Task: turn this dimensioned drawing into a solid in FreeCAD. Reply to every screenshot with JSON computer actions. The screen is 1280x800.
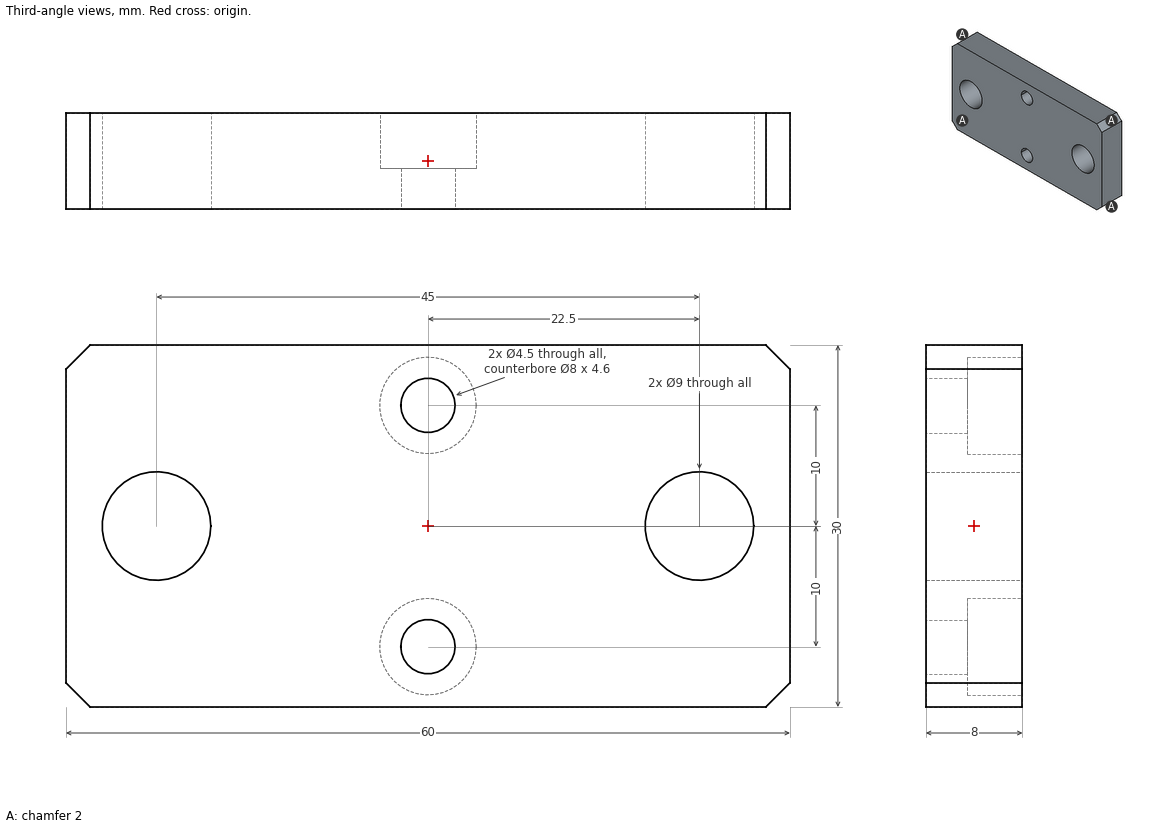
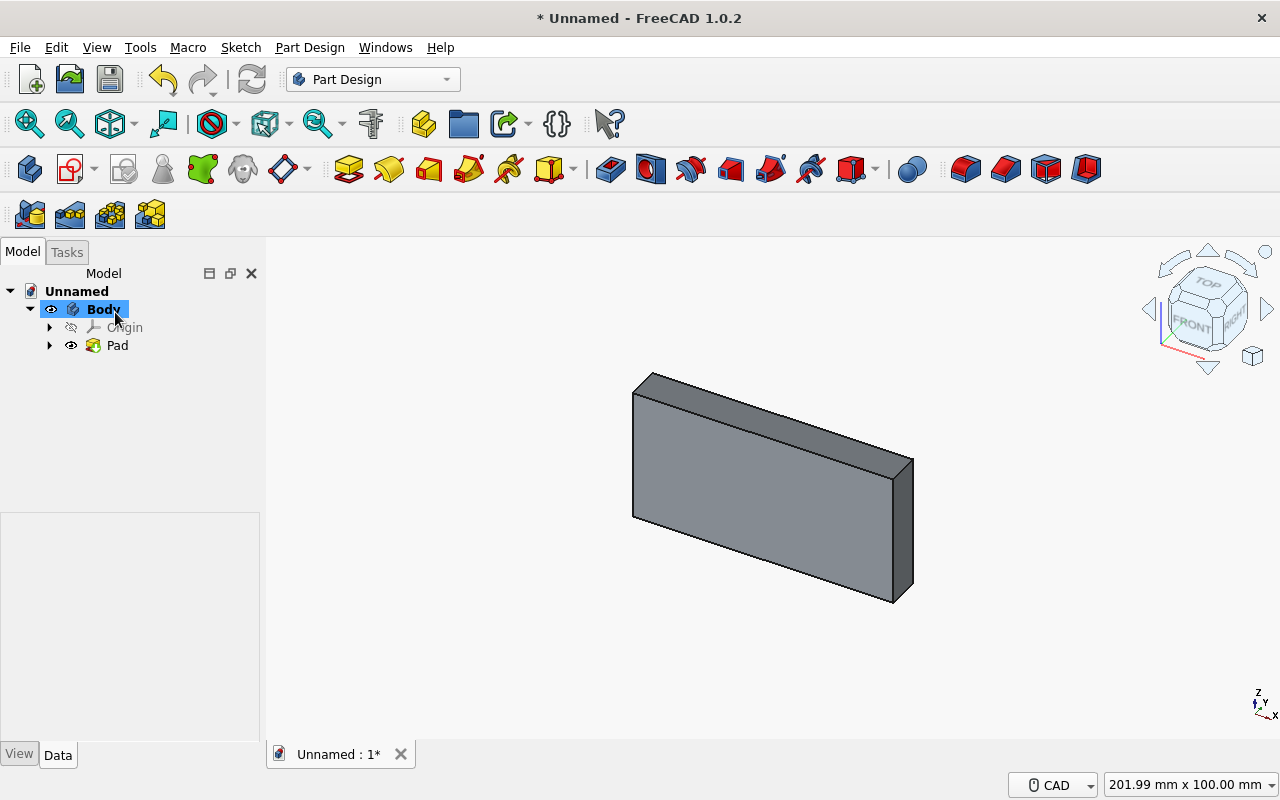
{"action": "left_click", "coordinate": [903, 469]}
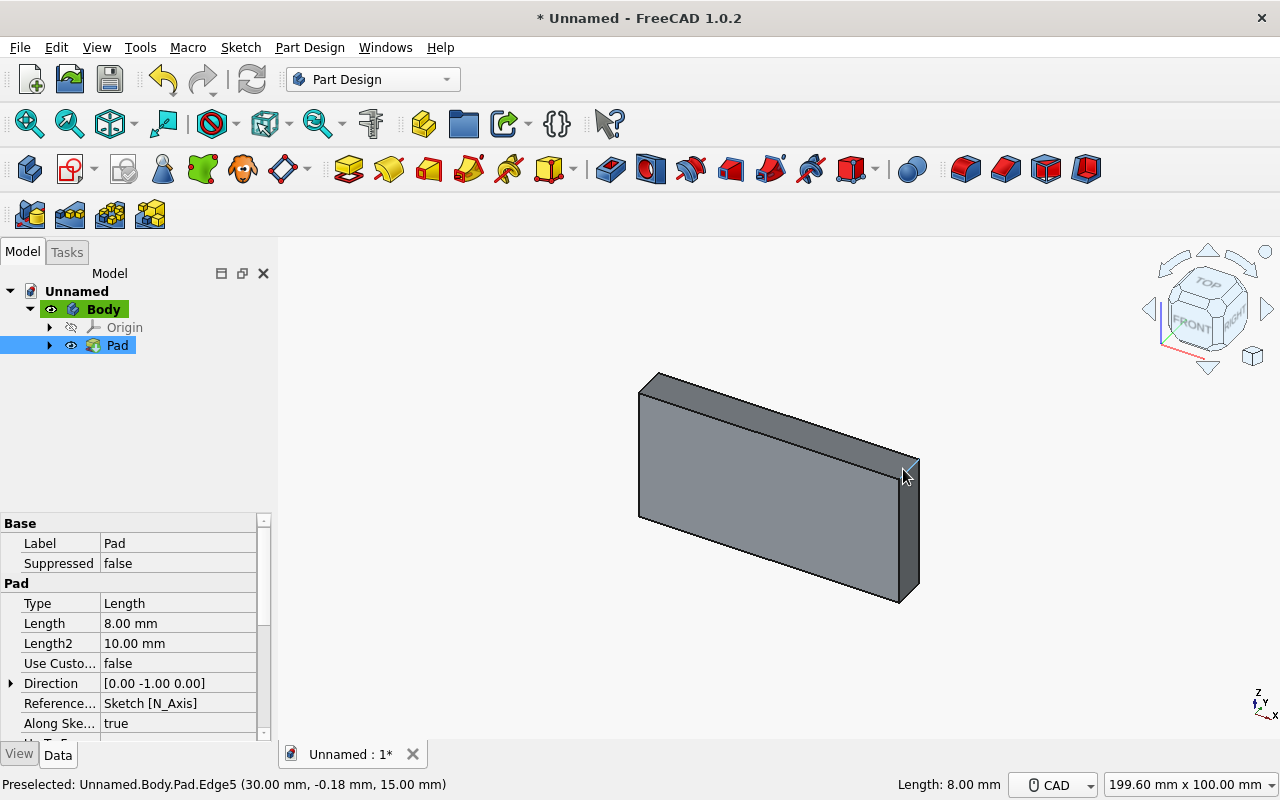
{"action": "key", "text": "0"}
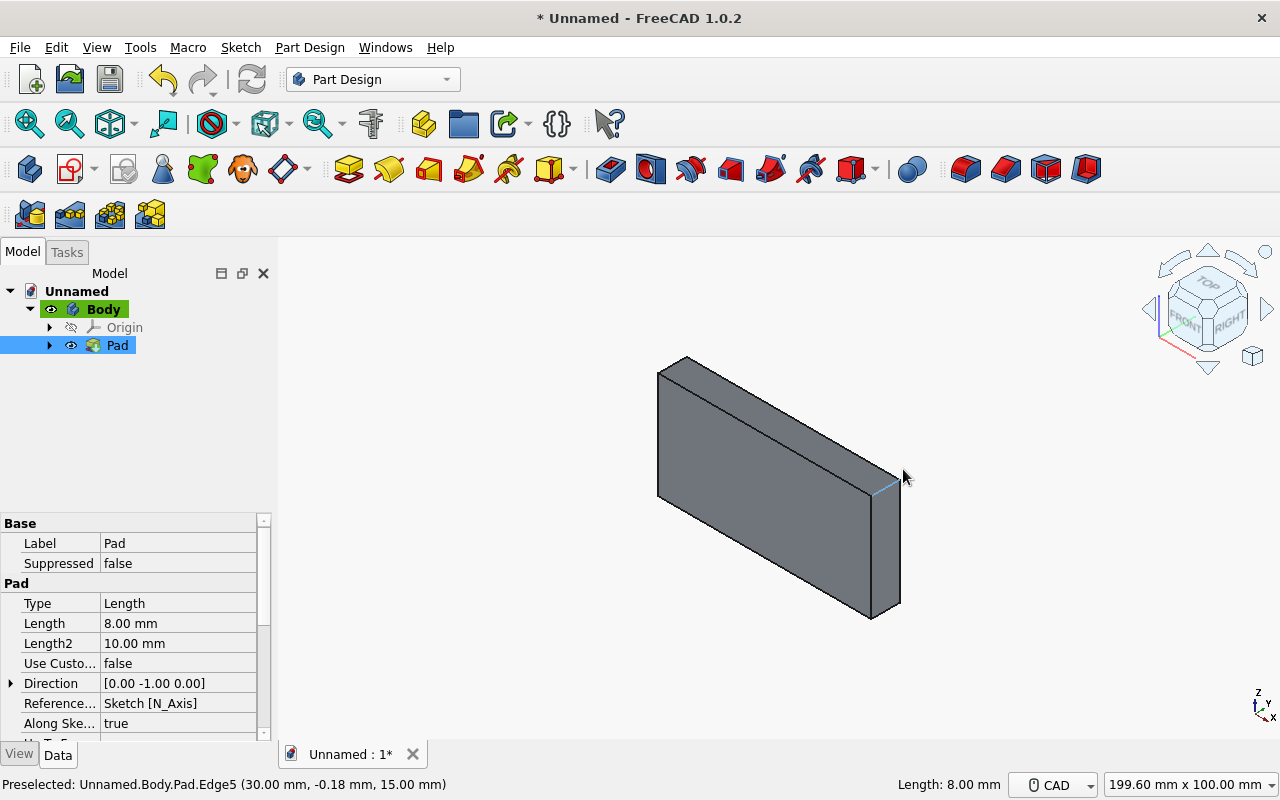
{"action": "key", "text": "2"}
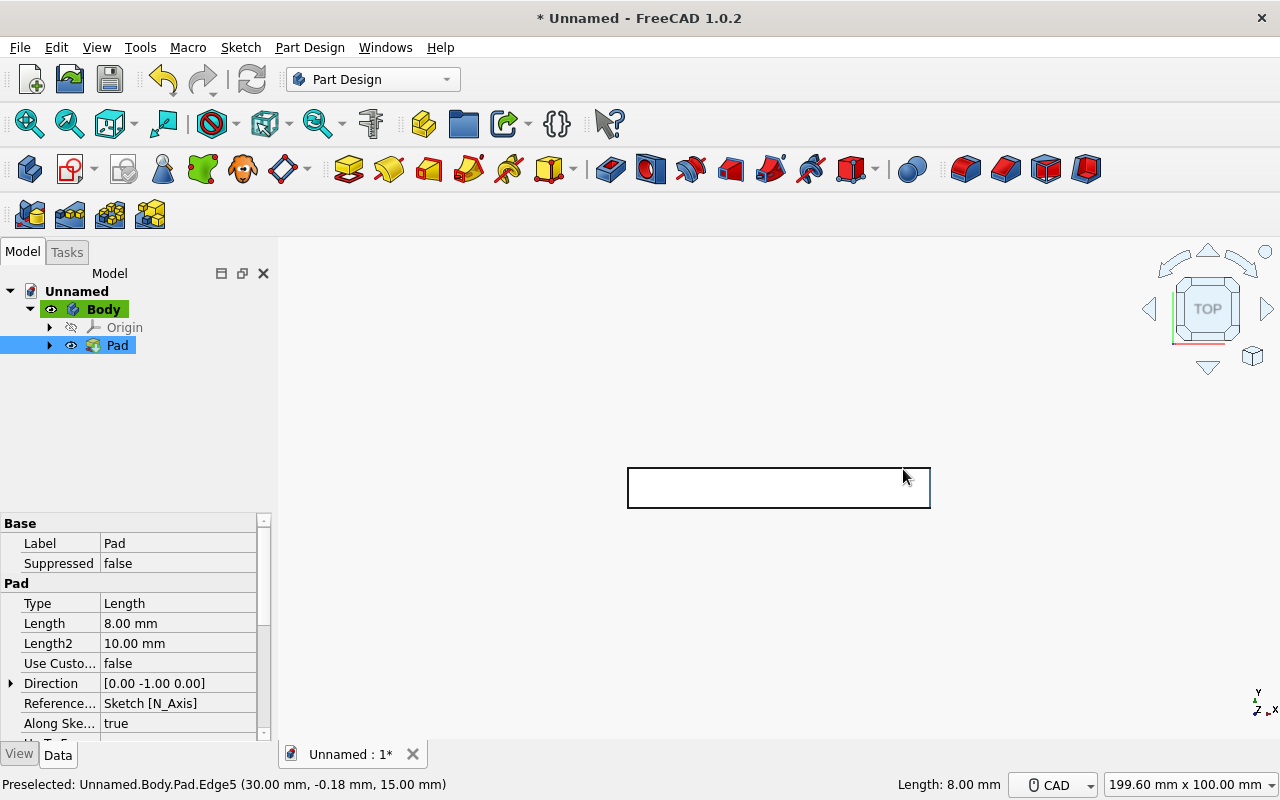
{"action": "left_click", "coordinate": [30, 124]}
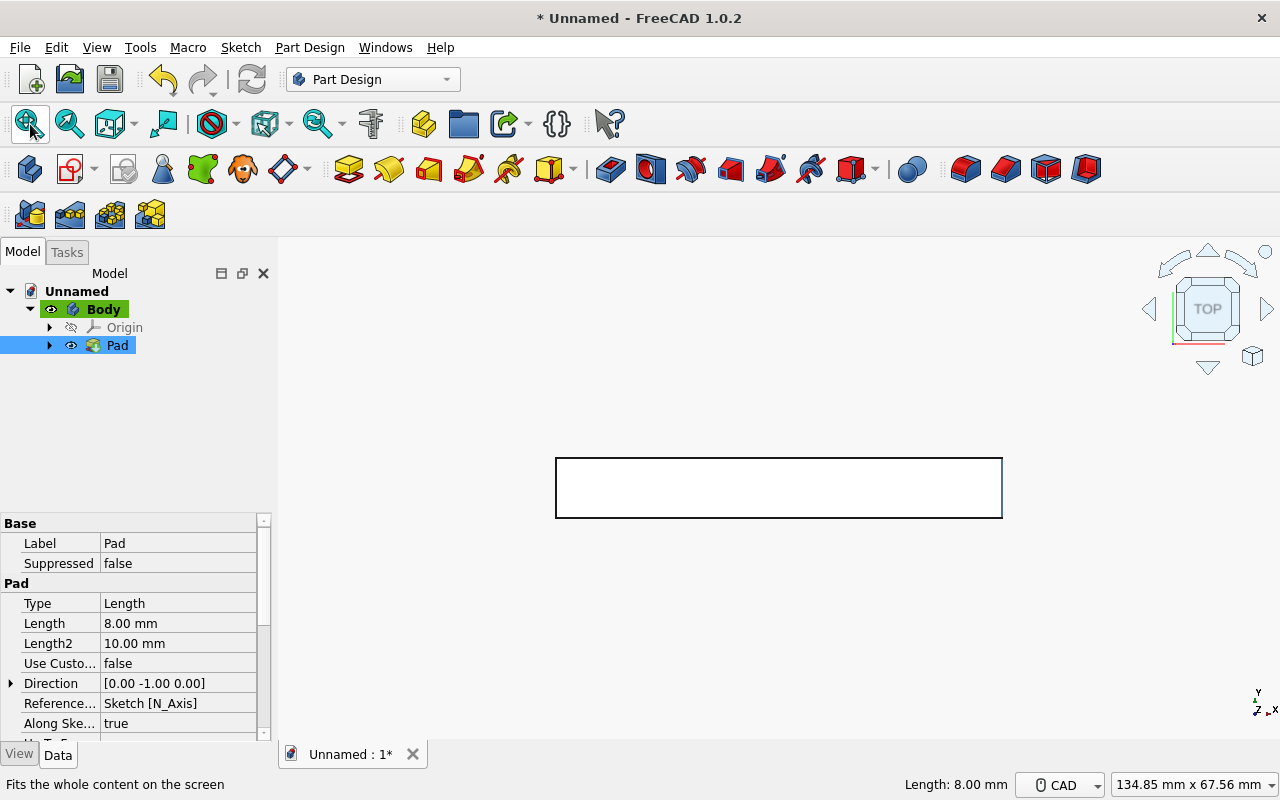
{"action": "left_click", "coordinate": [556, 487], "text": "ctrl"}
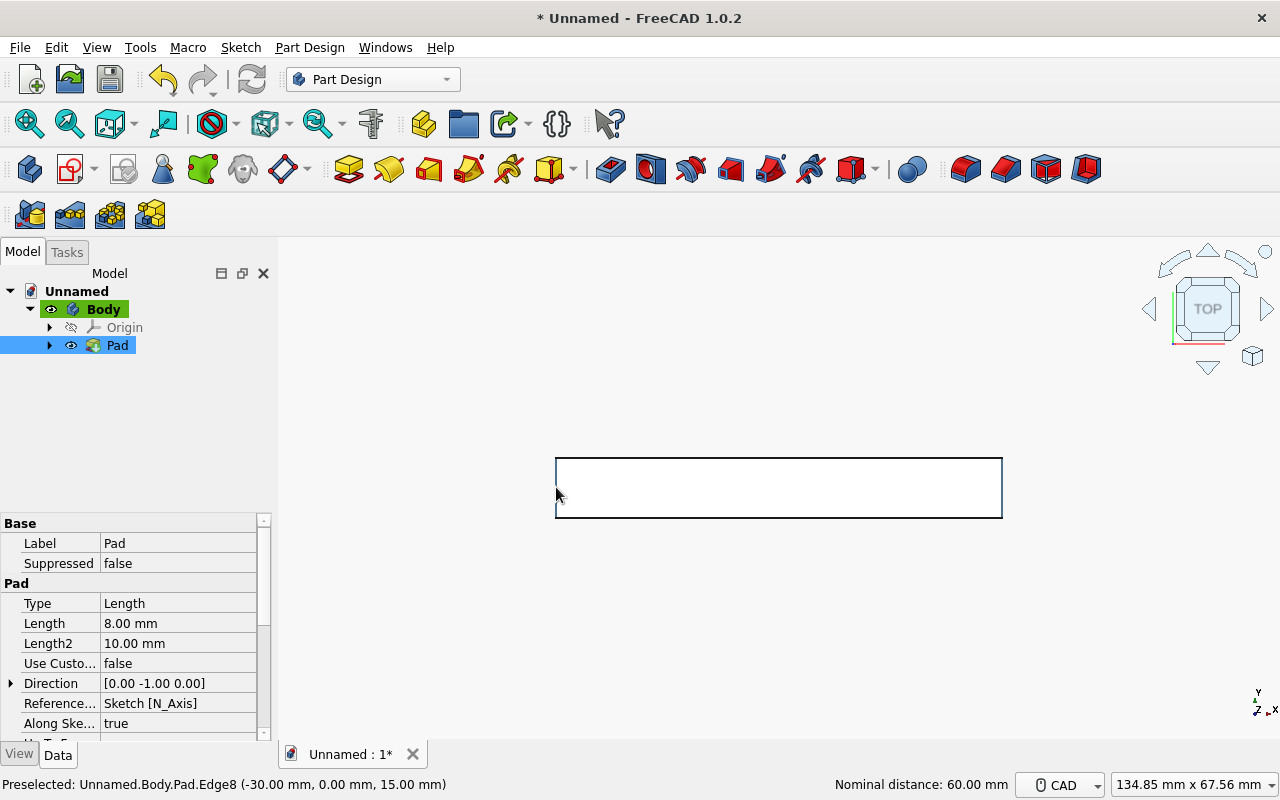
{"action": "key", "text": "1"}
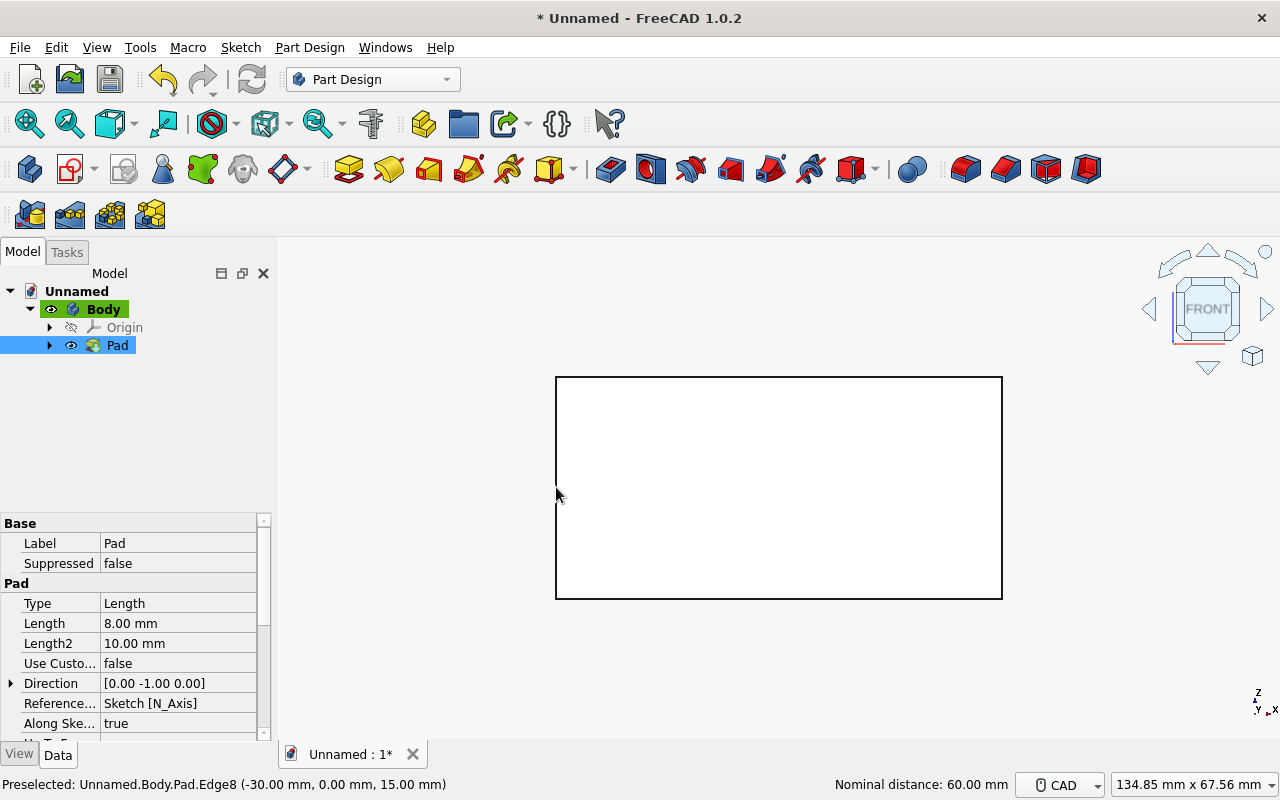
{"action": "left_click", "coordinate": [30, 124]}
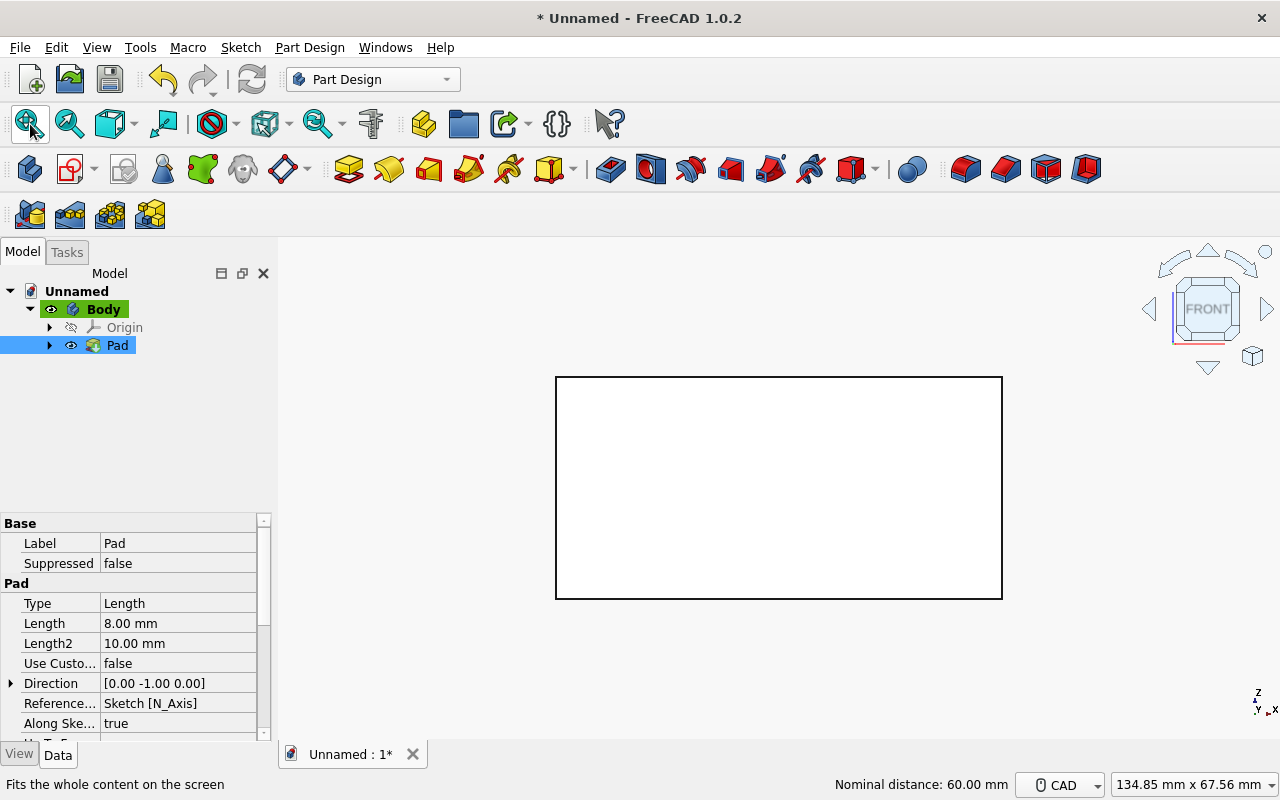
{"action": "key", "text": "3"}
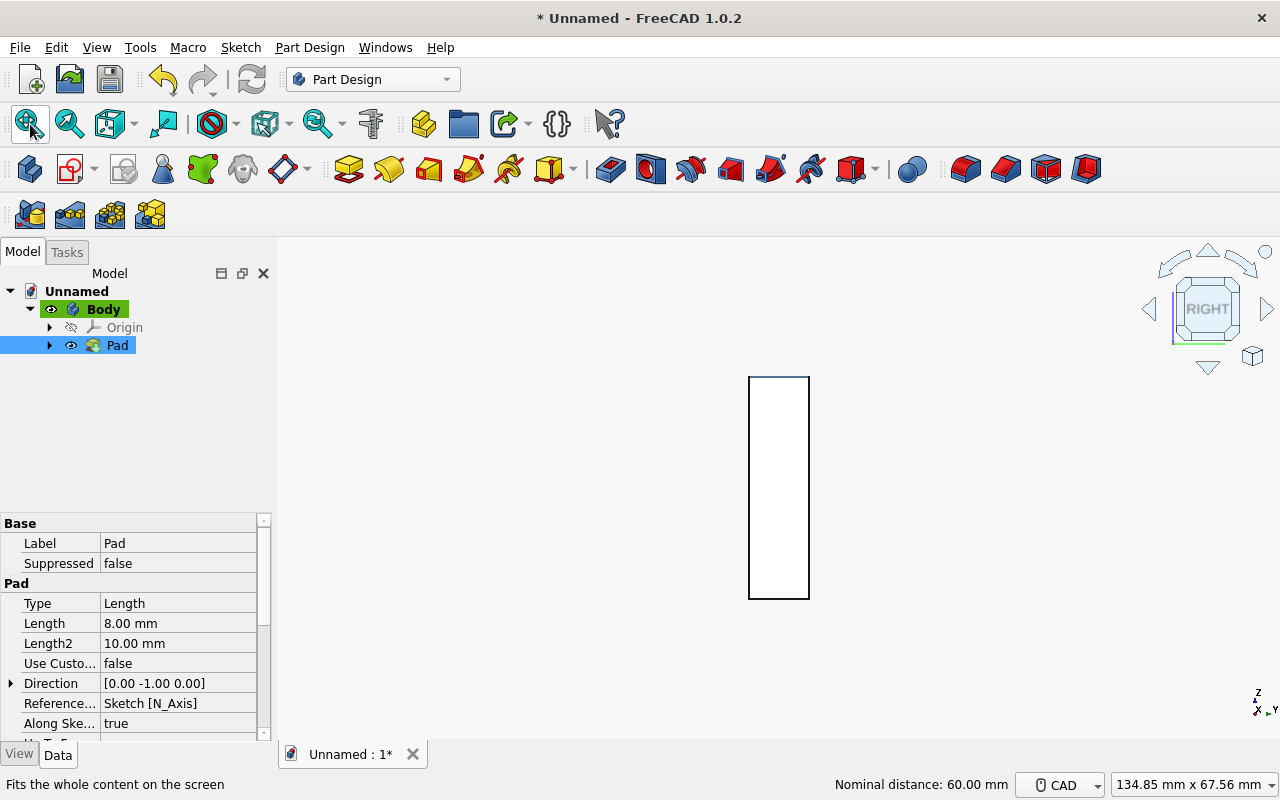
{"action": "left_click", "coordinate": [30, 124]}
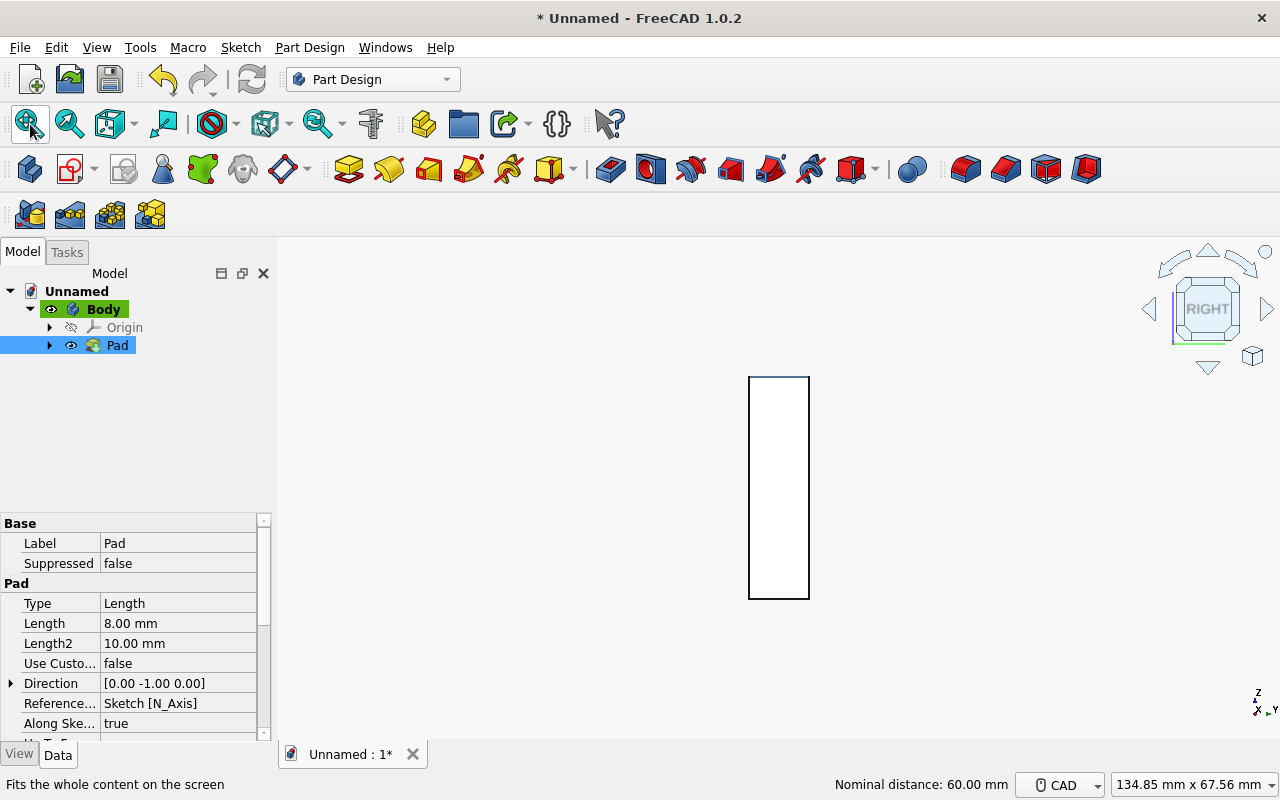
{"action": "left_click", "coordinate": [779, 598], "text": "ctrl"}